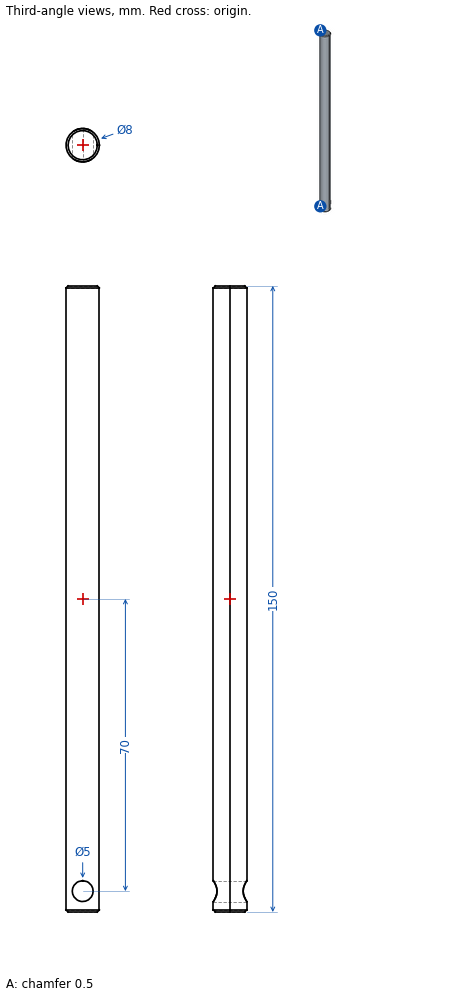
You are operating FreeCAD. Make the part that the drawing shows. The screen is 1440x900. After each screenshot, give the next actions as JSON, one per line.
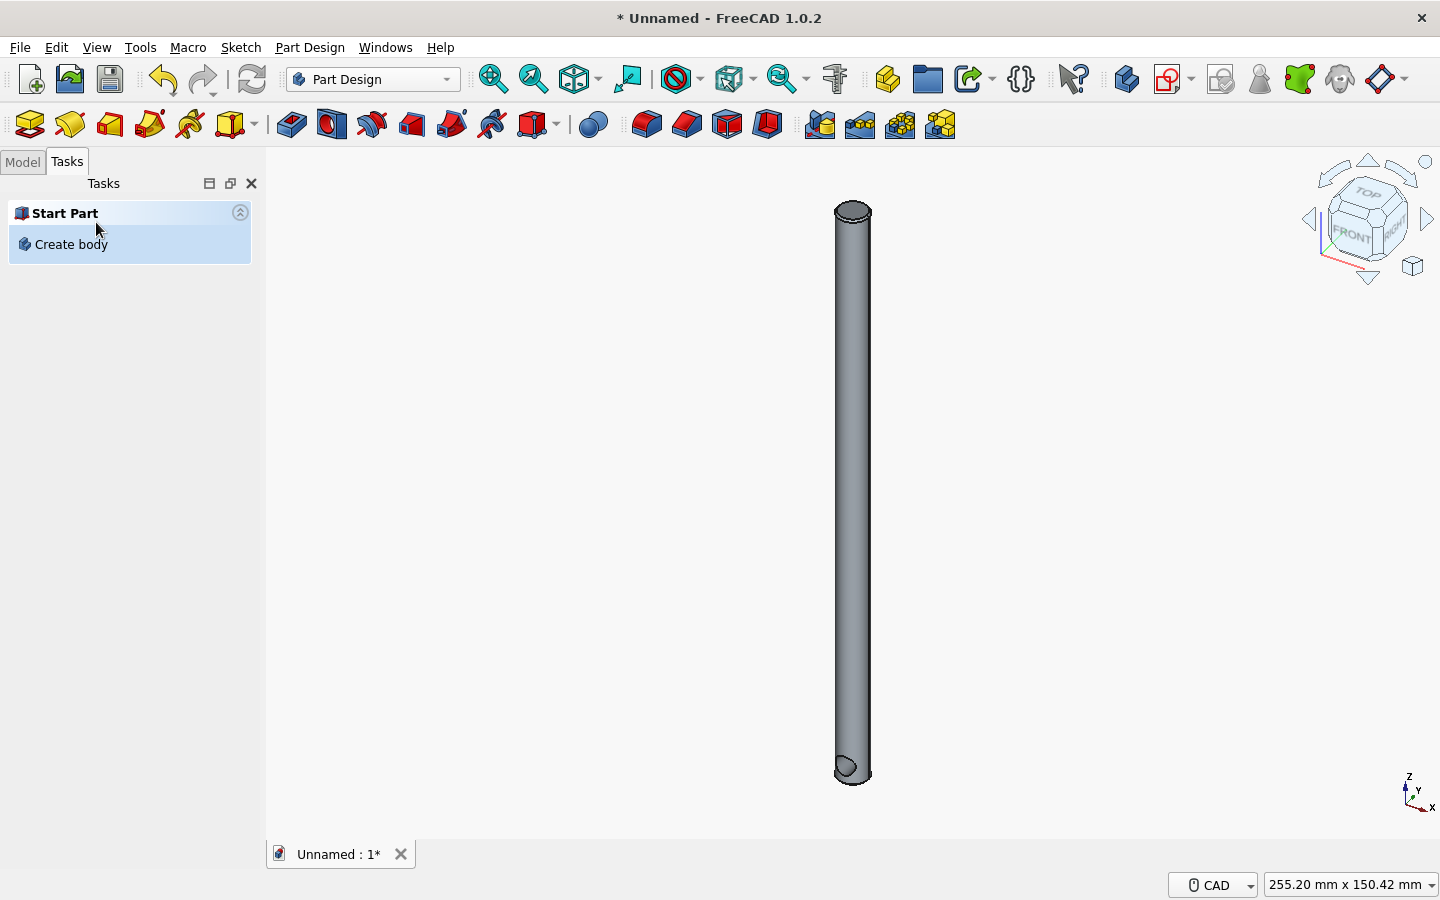
{"action": "key", "text": "0"}